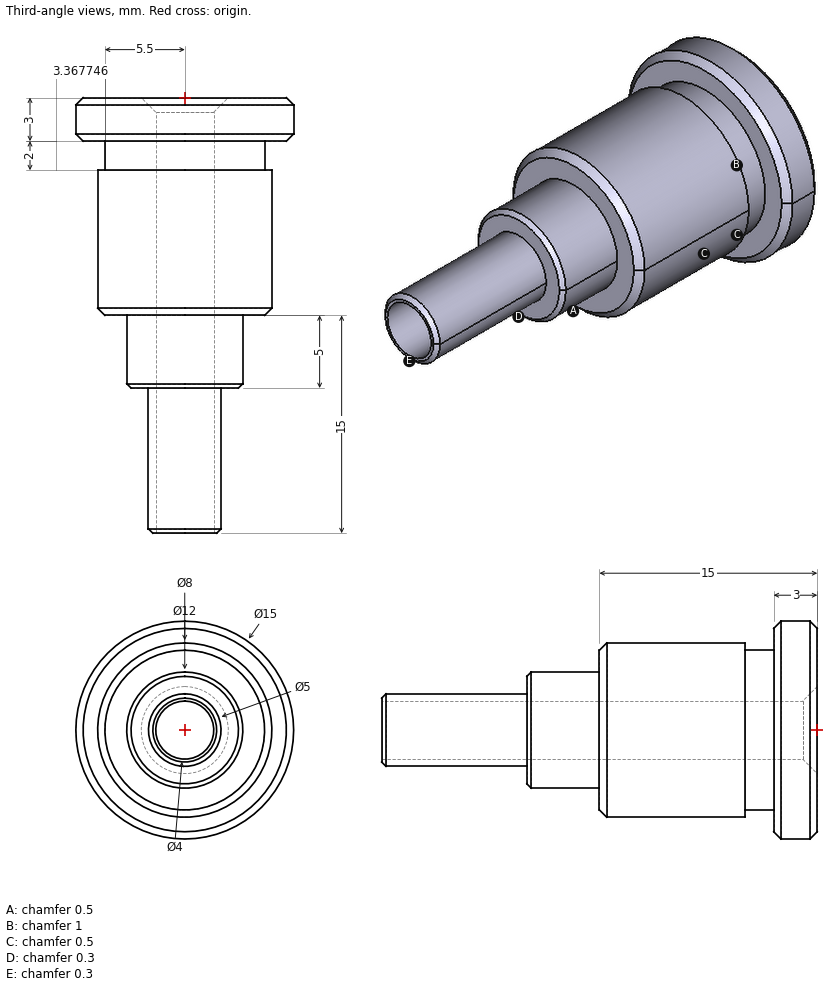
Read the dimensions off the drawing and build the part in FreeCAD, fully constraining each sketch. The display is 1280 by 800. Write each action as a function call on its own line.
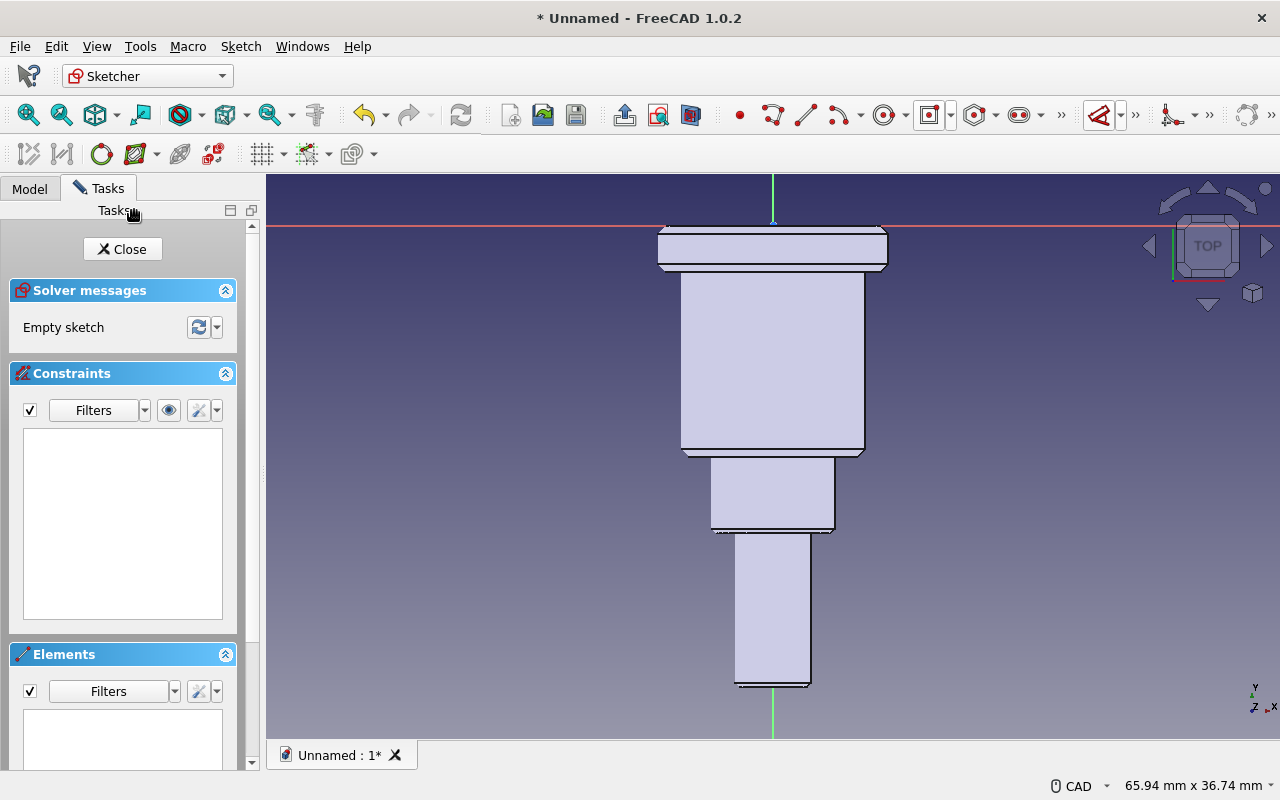
key(q)
key(s)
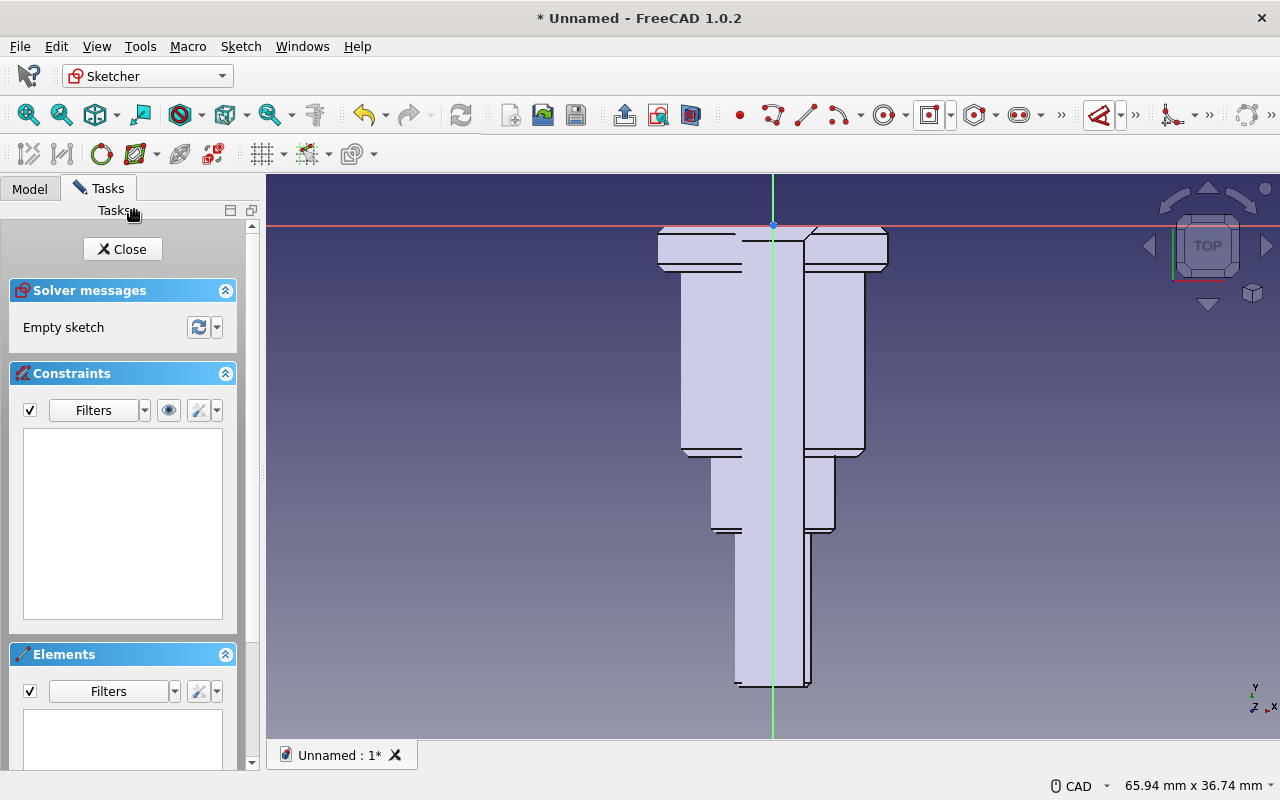
scroll(658, 270, up, 12)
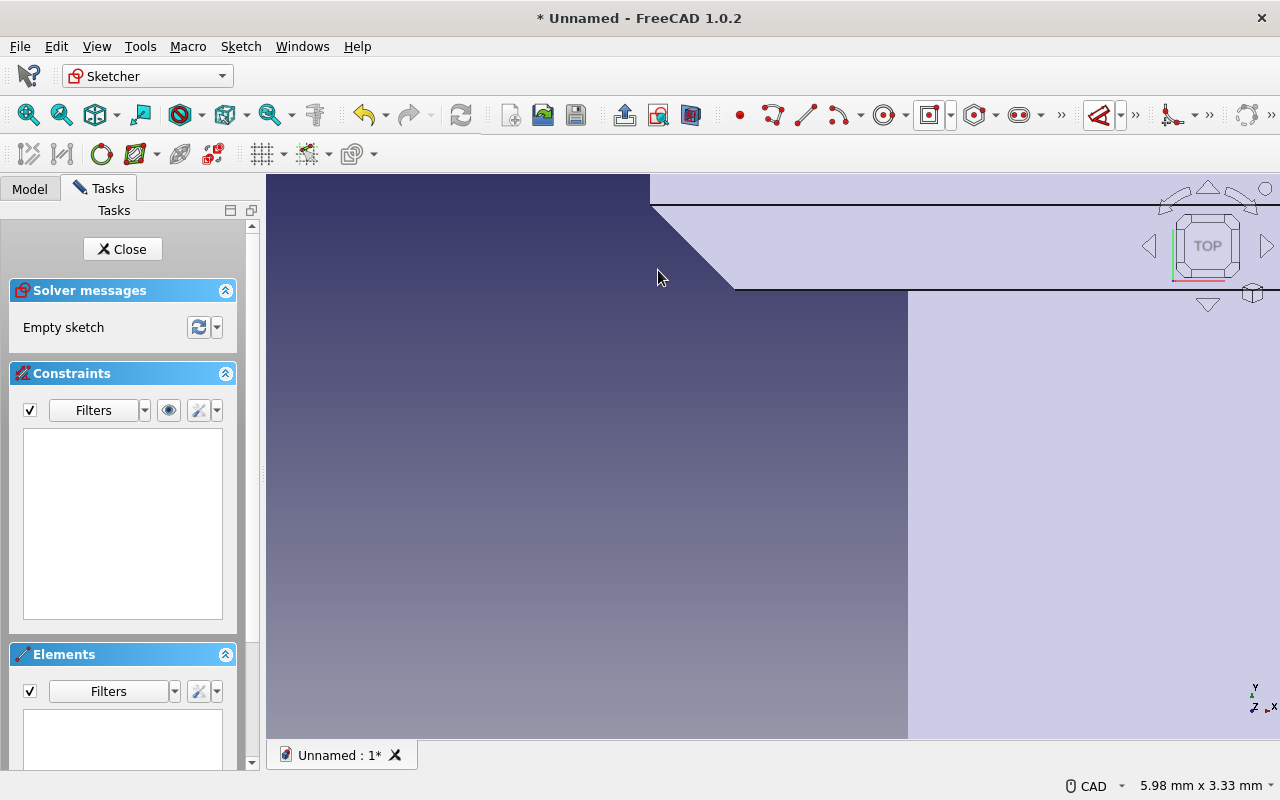
click(950, 116)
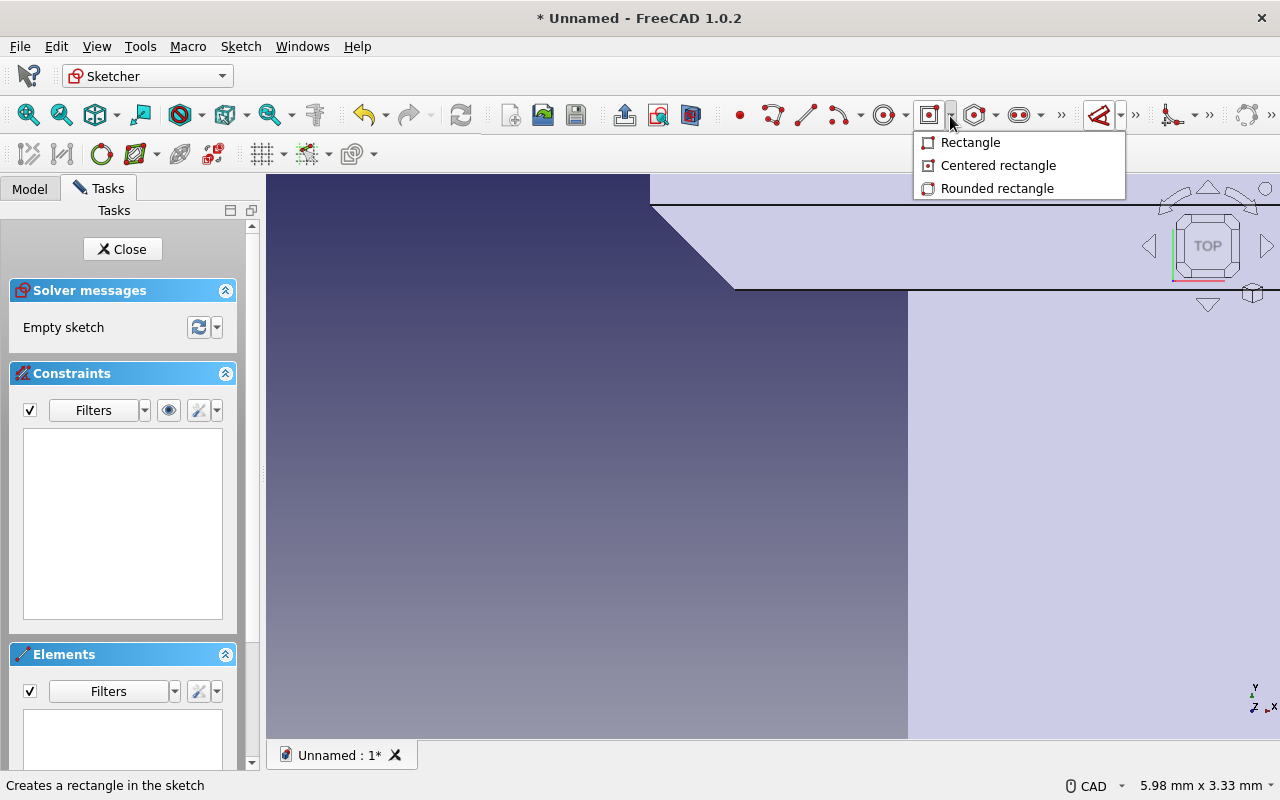
click(1020, 142)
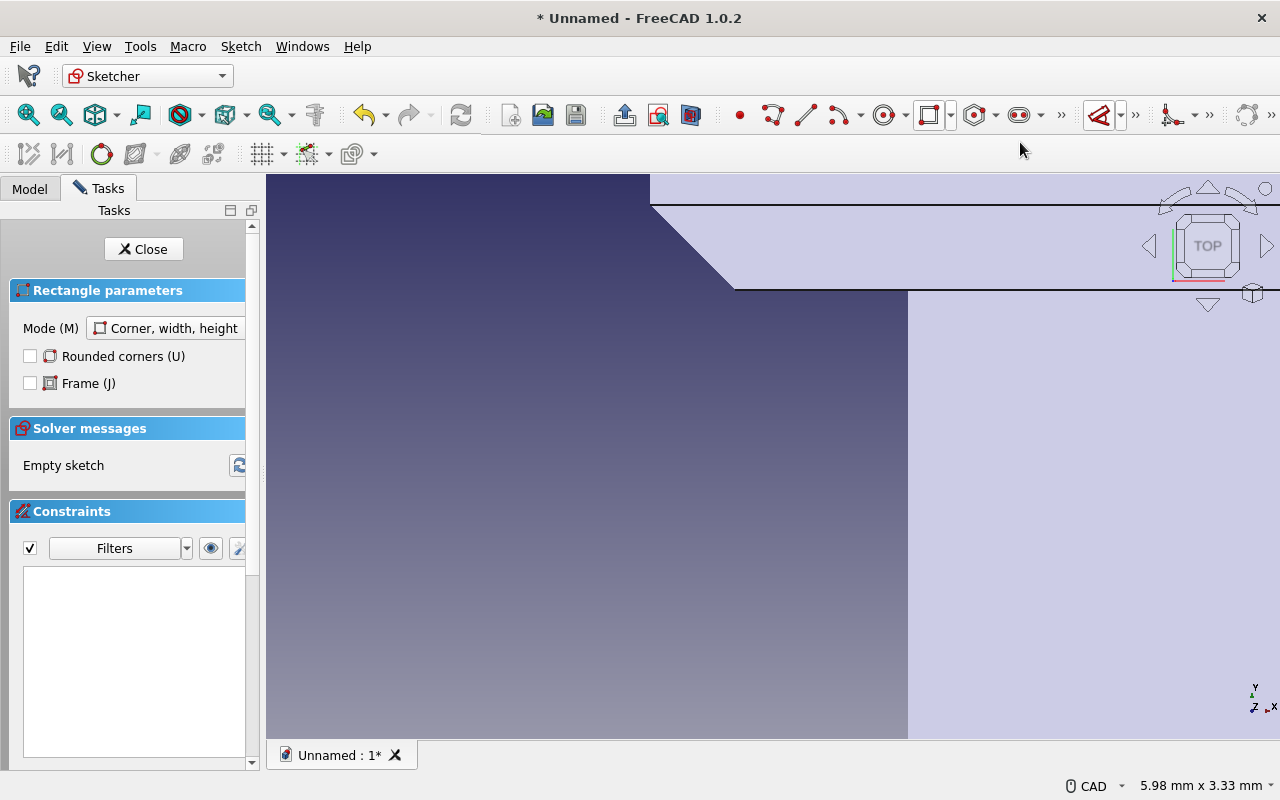
click(419, 290)
move(989, 629)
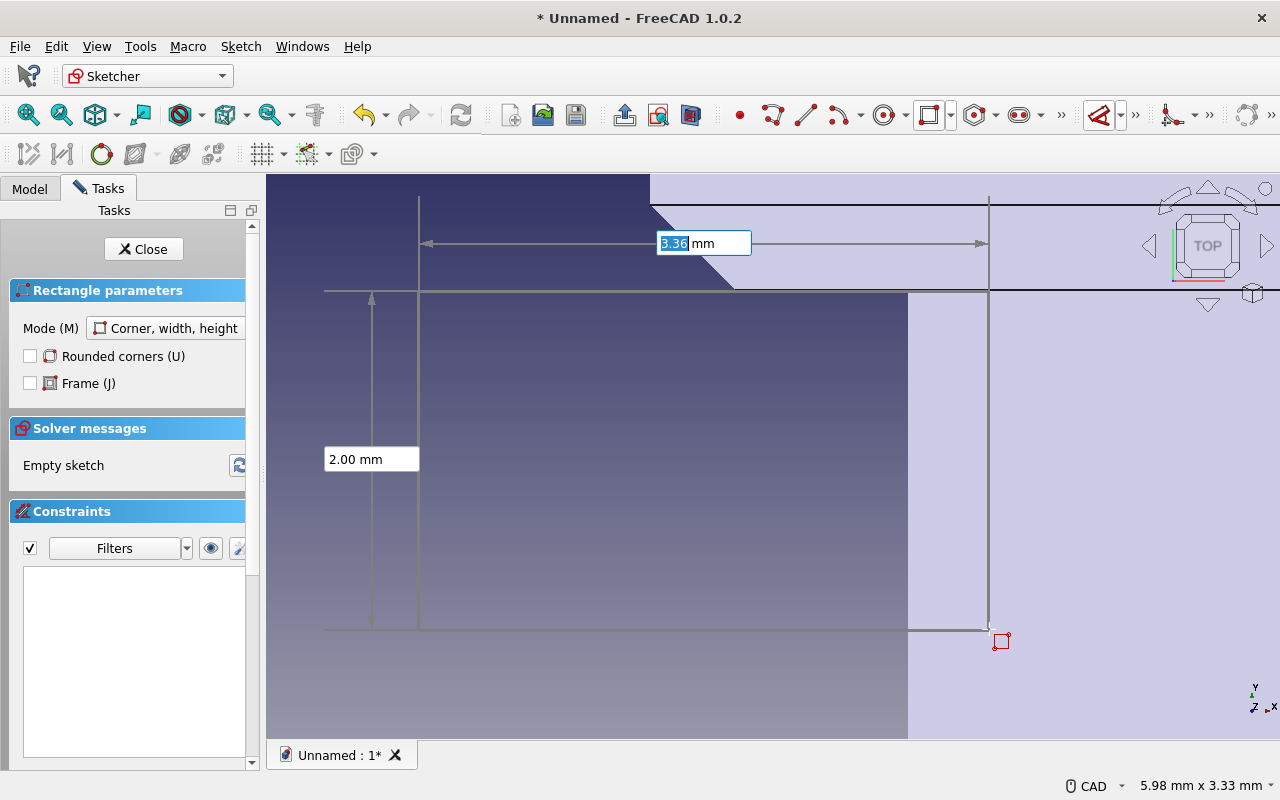
text(3.367746)
key(Tab)
text(2)
key(Return)
key(Escape)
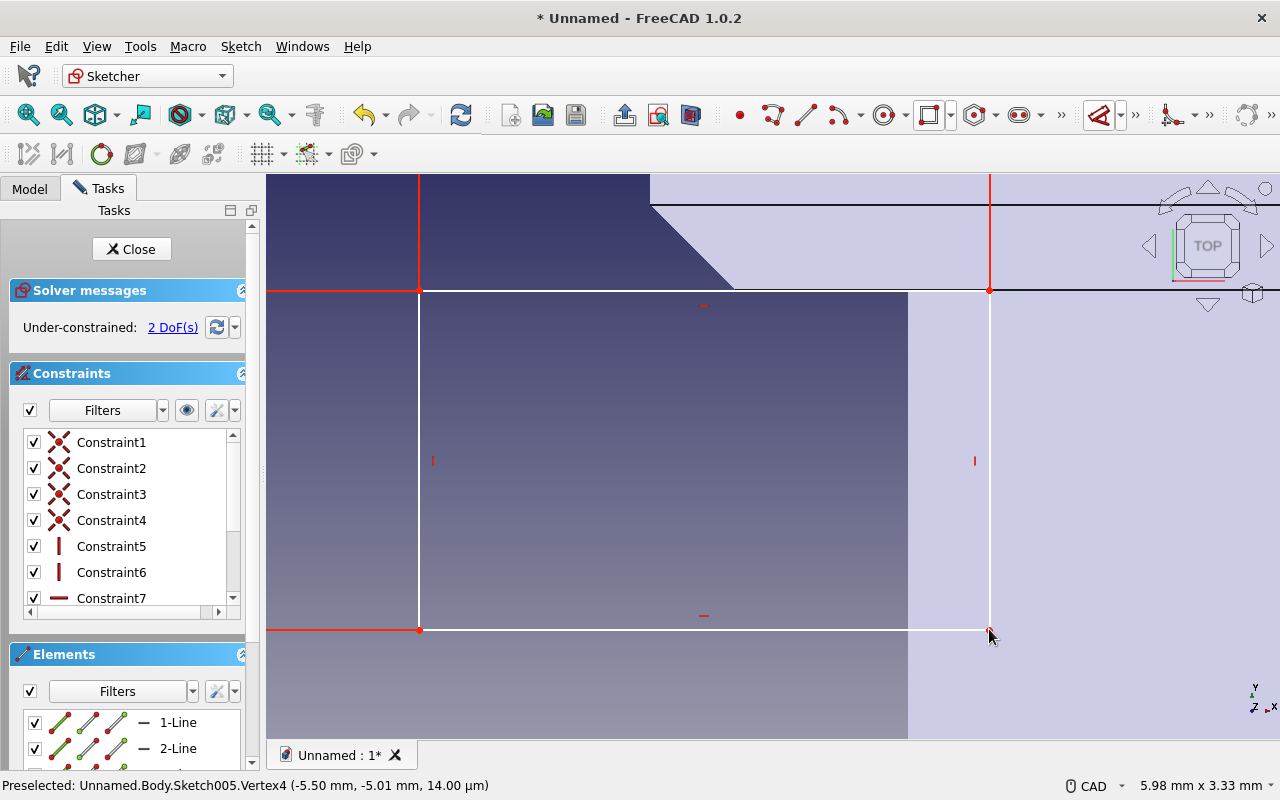
click(419, 291)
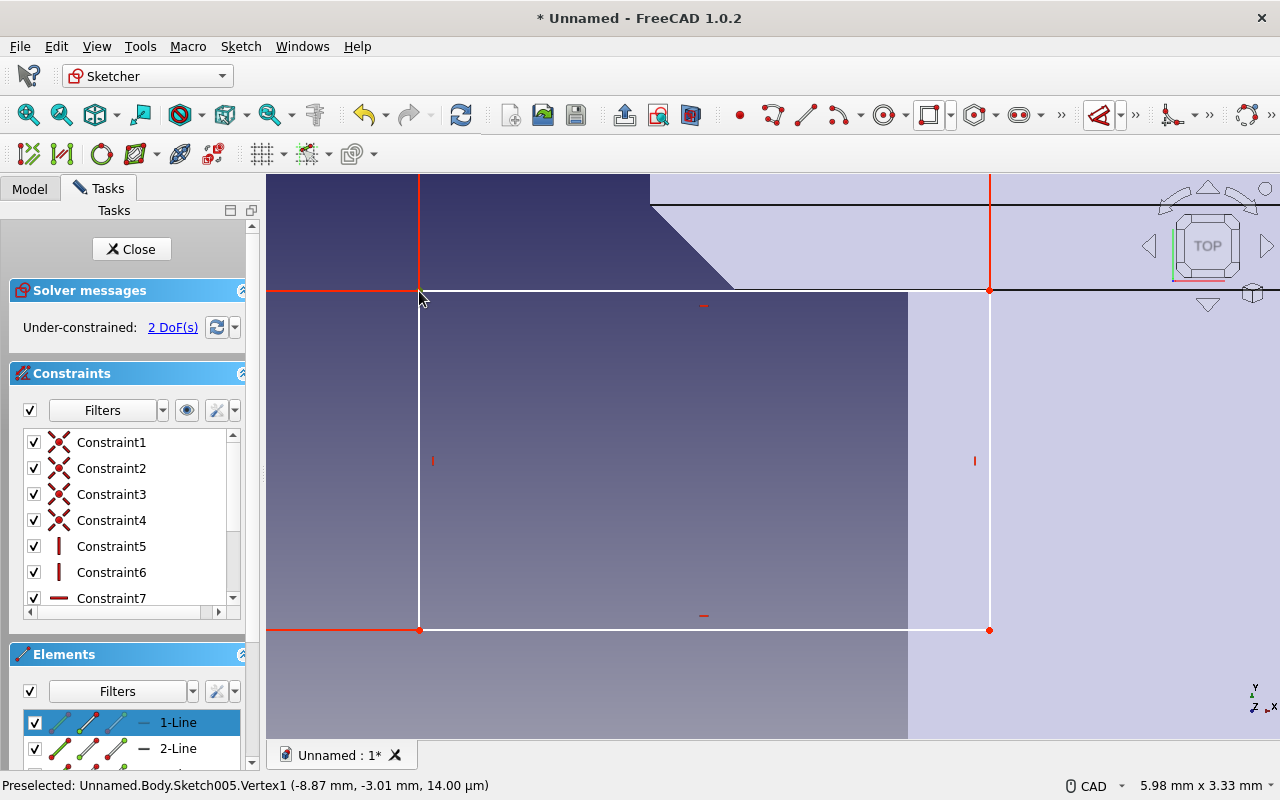
click(1120, 116)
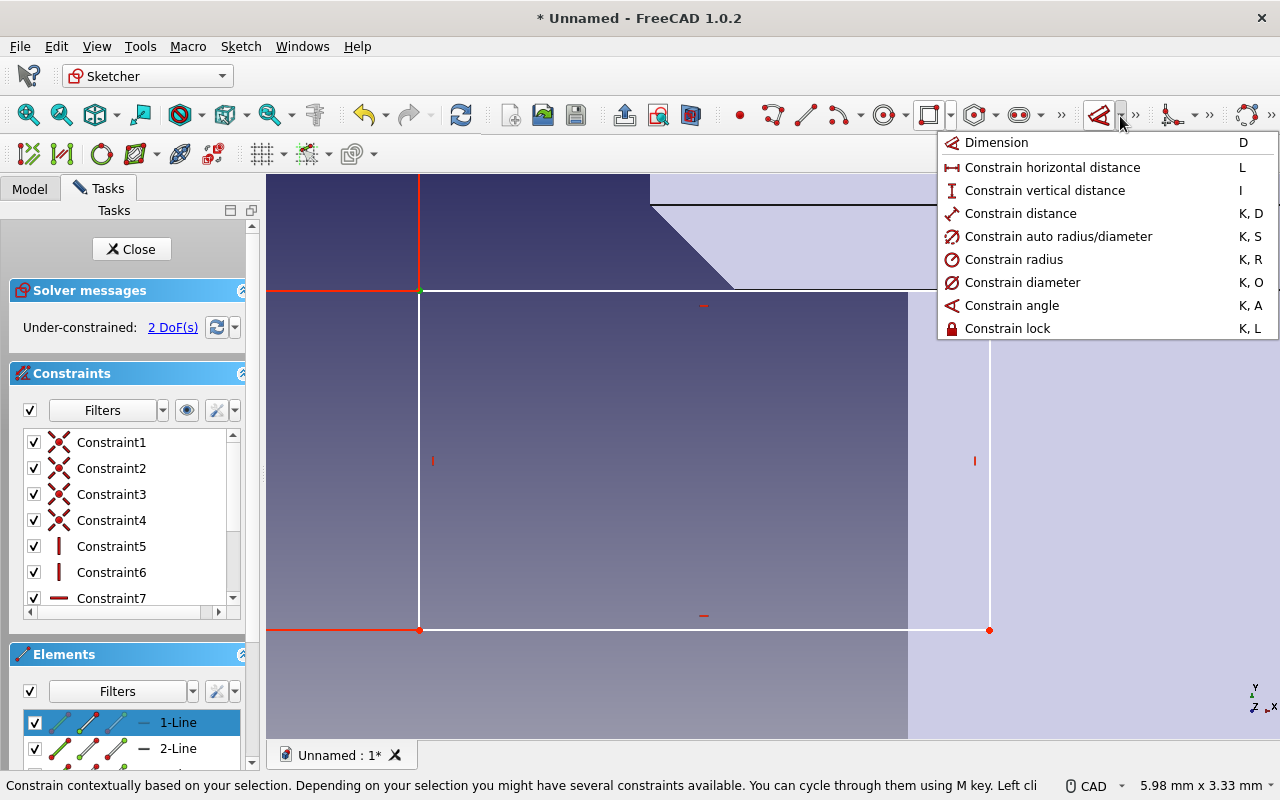
click(1108, 190)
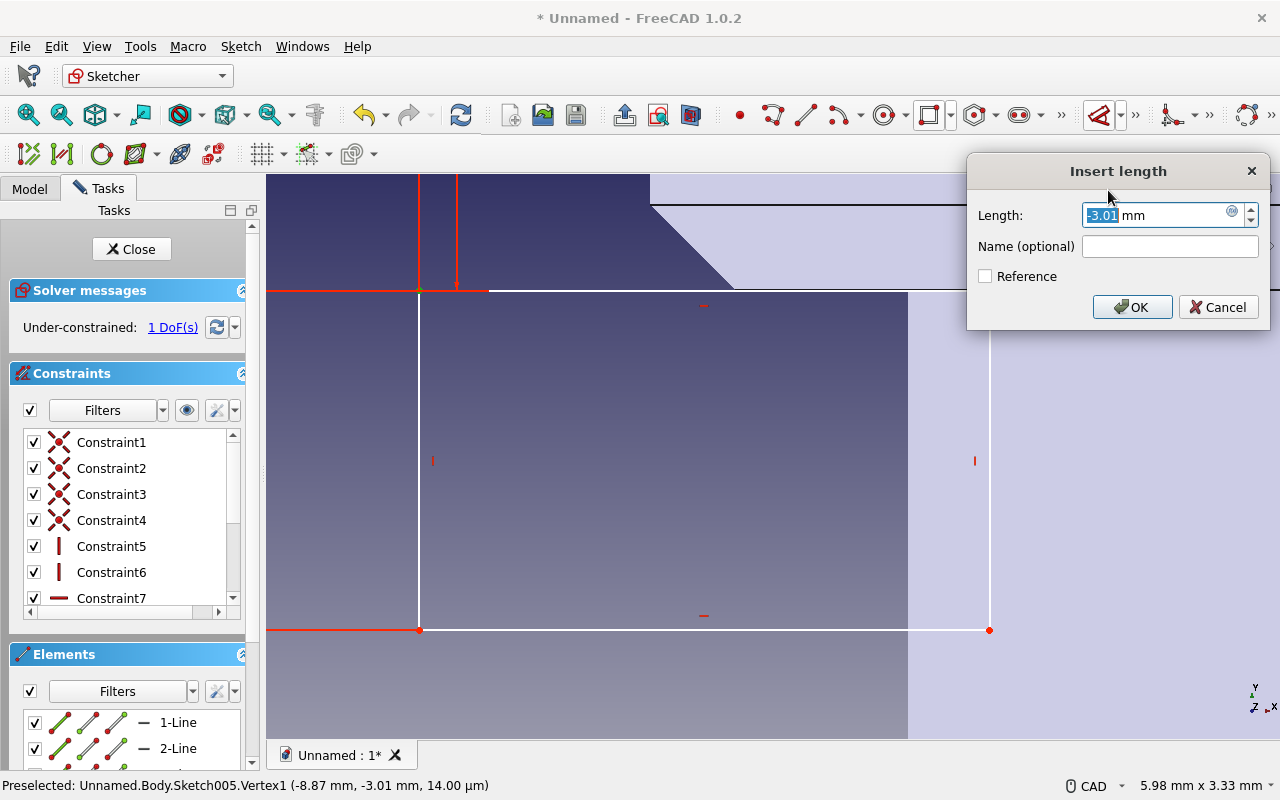
text(-3)
key(Return)